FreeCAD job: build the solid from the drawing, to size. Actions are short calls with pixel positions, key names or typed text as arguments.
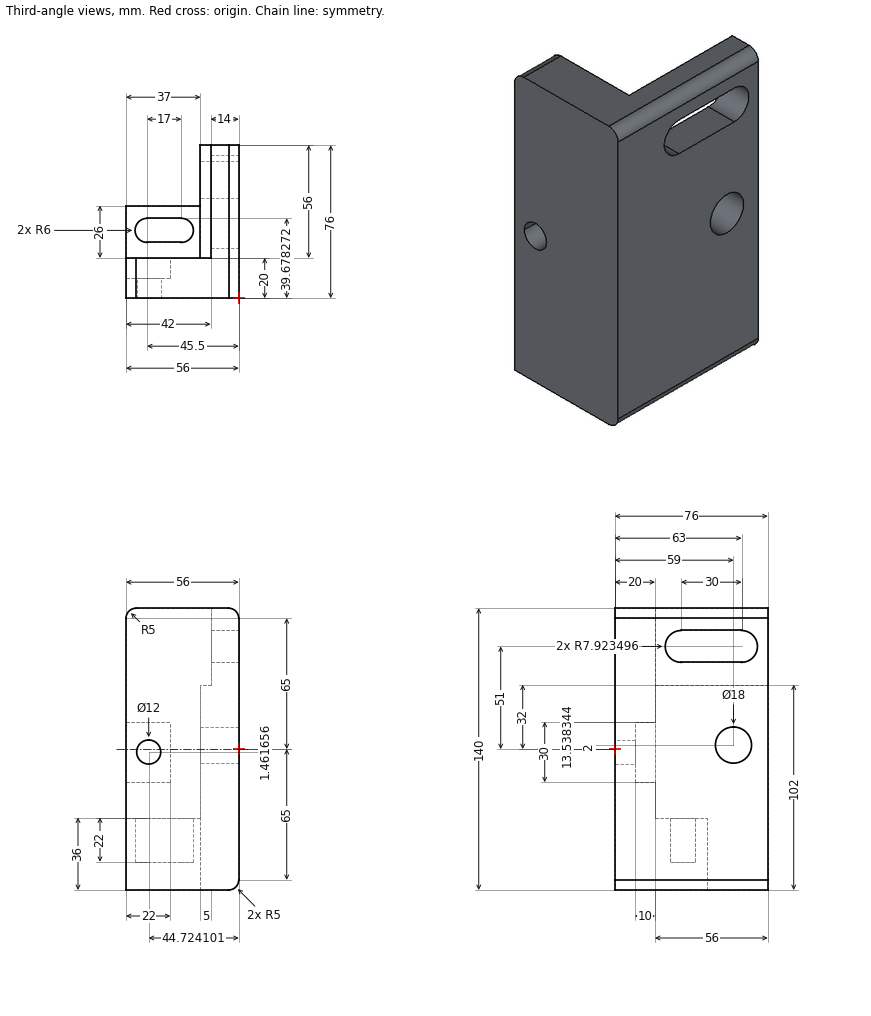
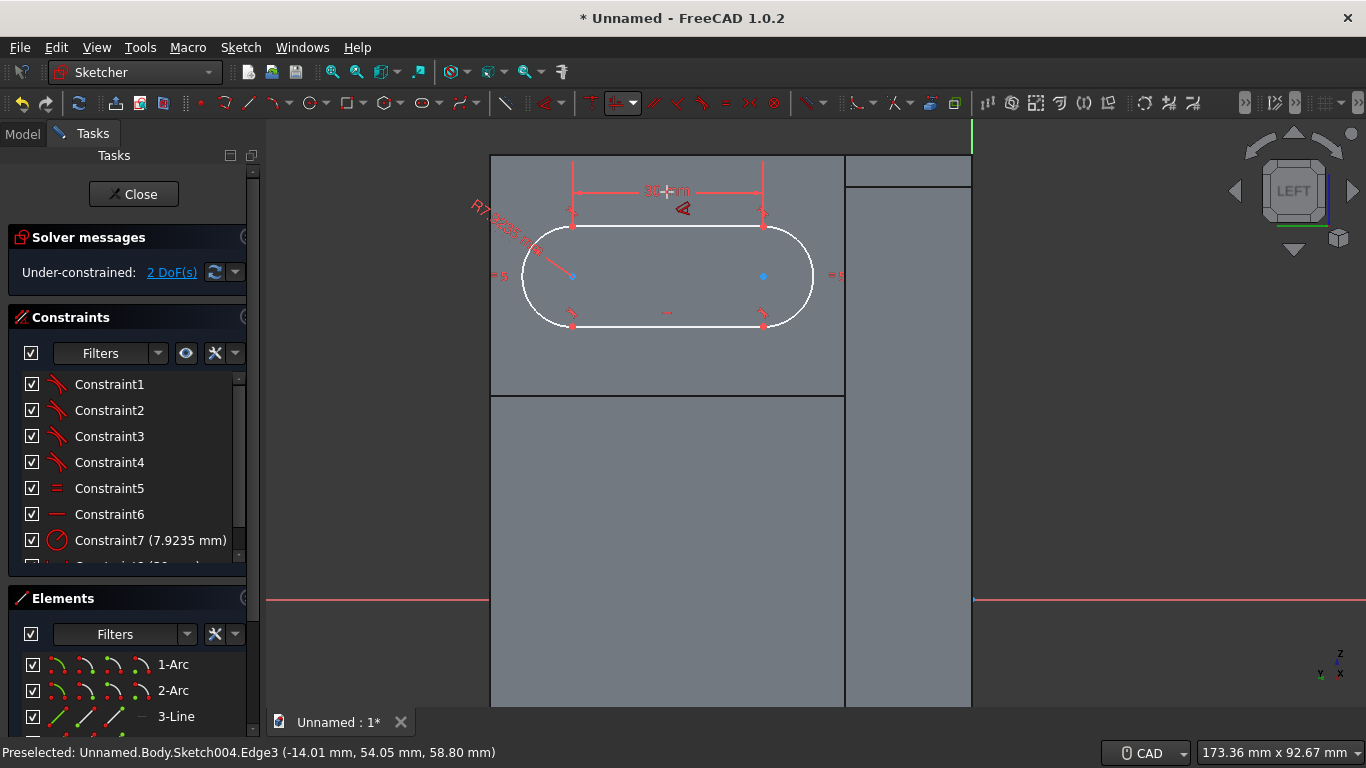
click(573, 226)
click(772, 634)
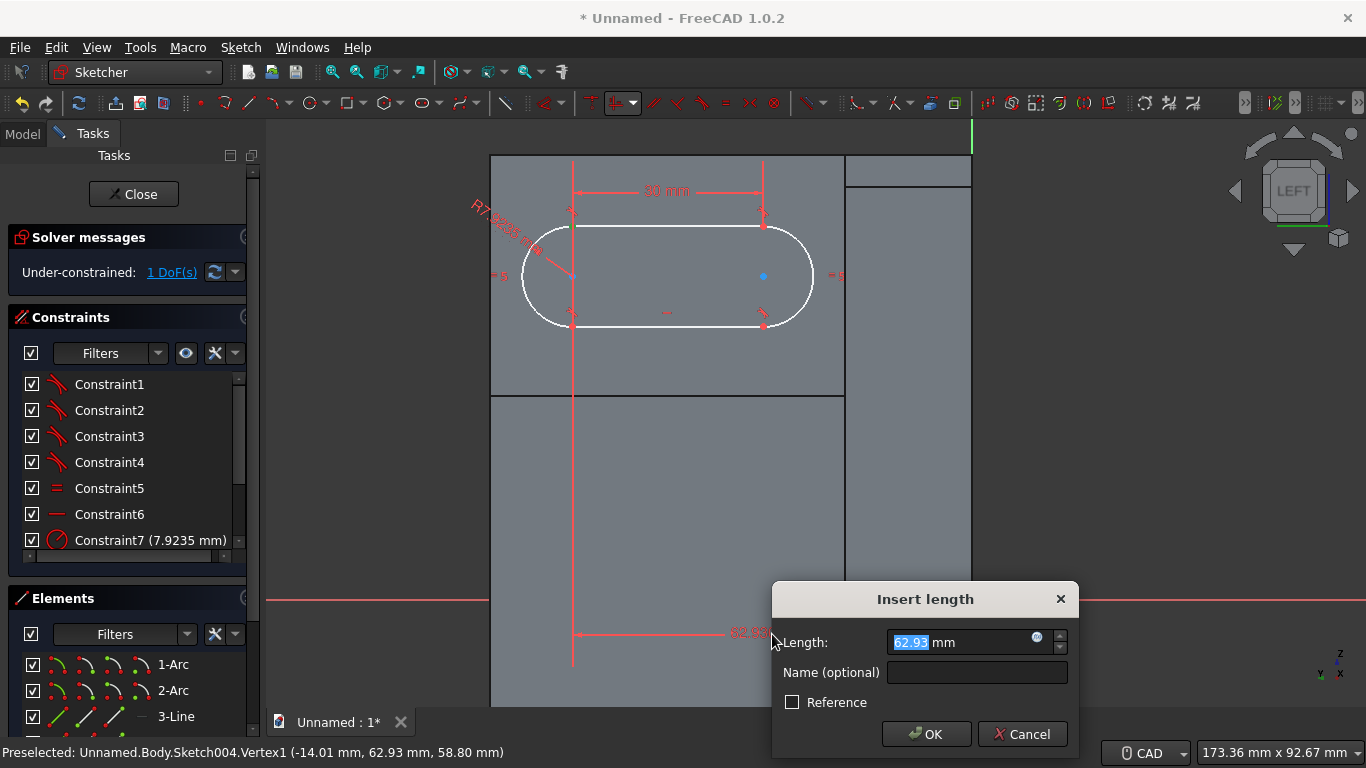
text(63)
key(Return)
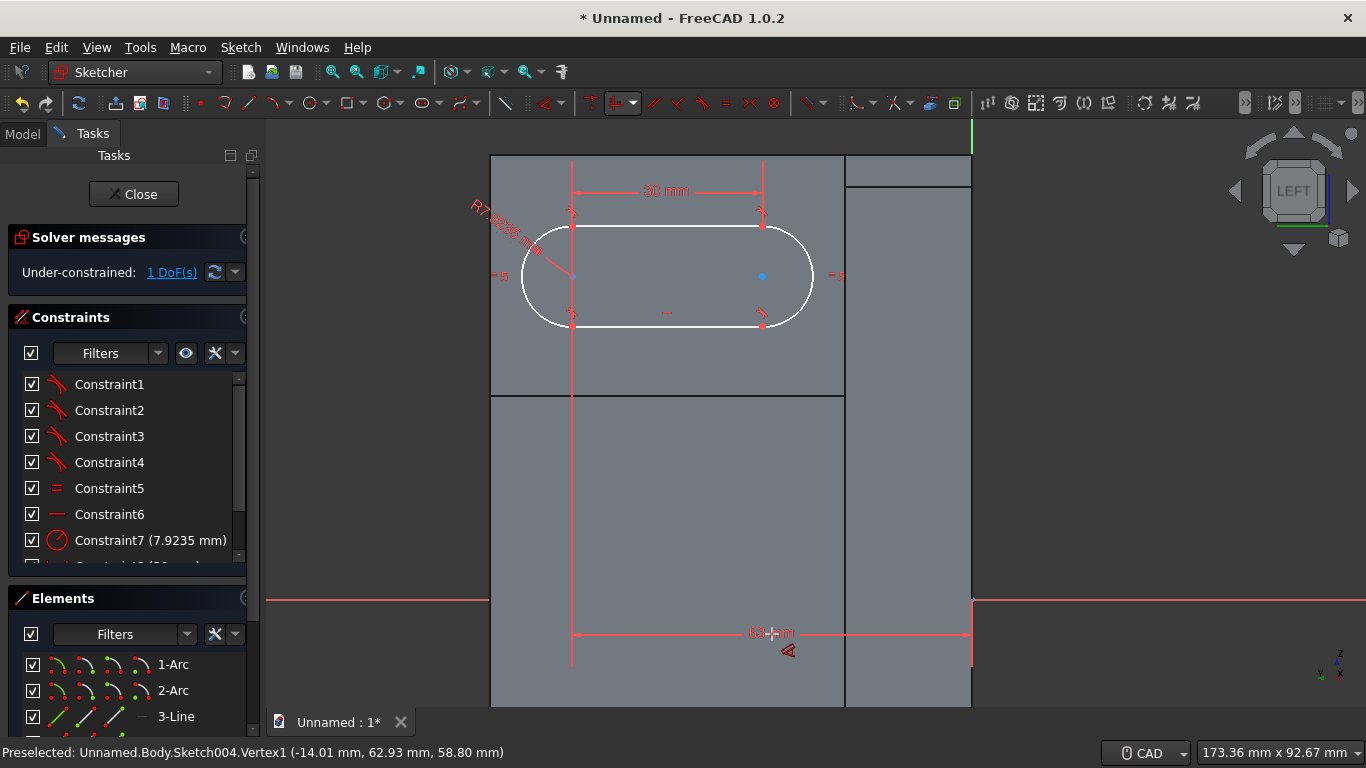
click(572, 277)
click(1006, 438)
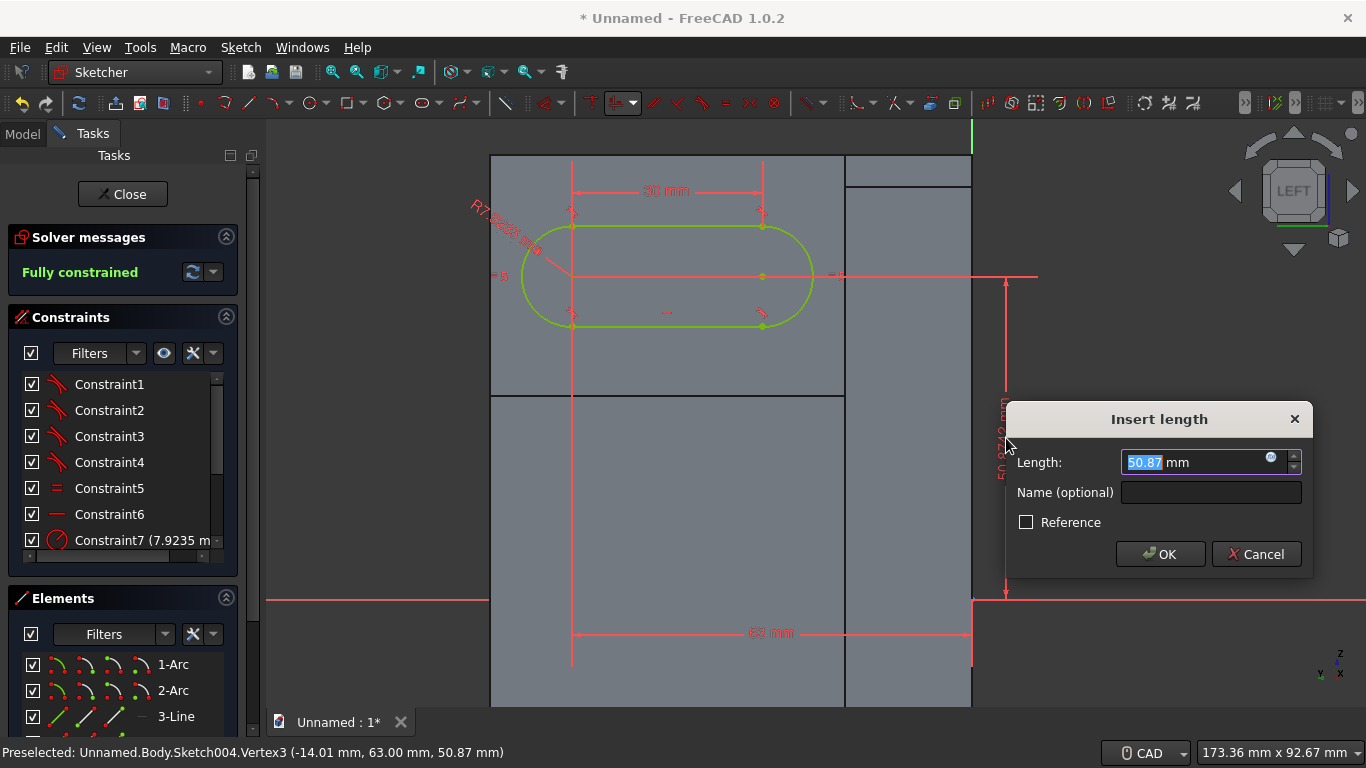
text(51)
key(Return)
key(Escape)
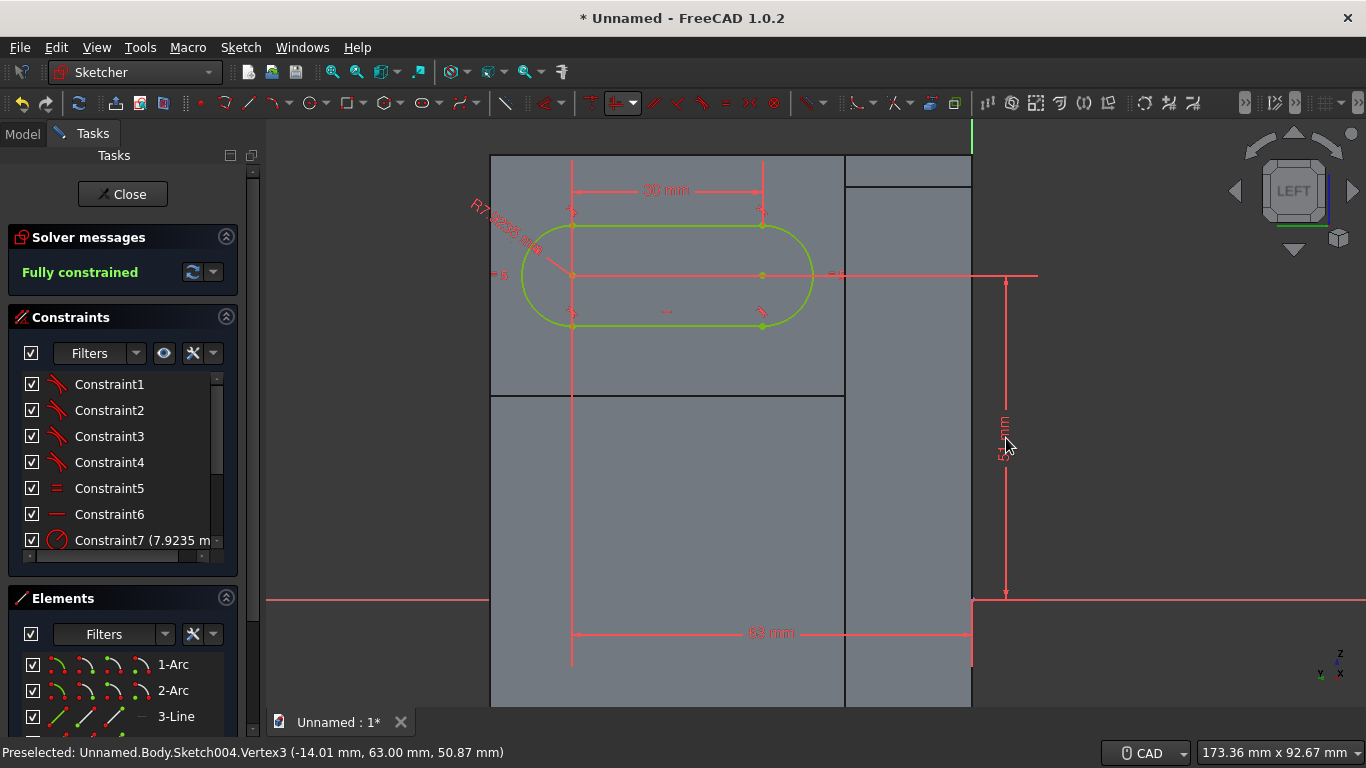
click(123, 194)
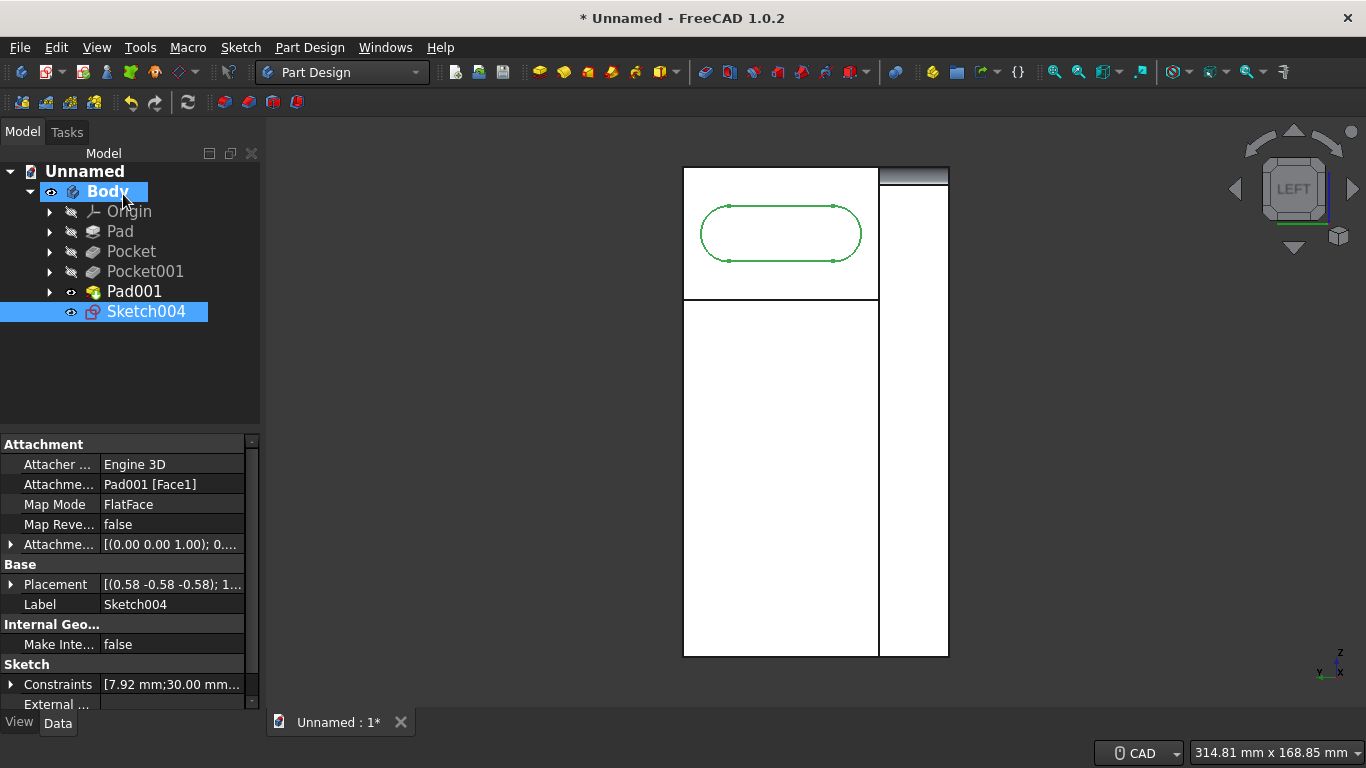
click(706, 72)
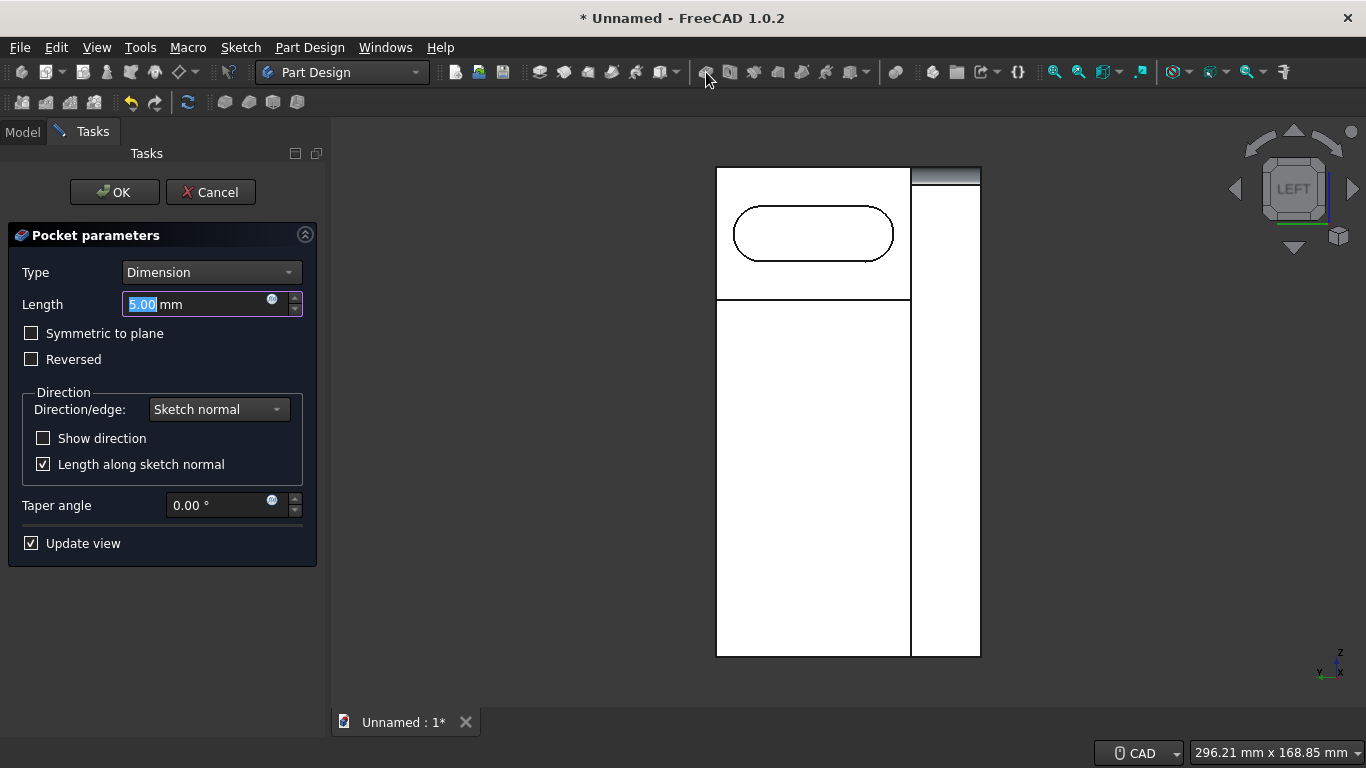
click(212, 272)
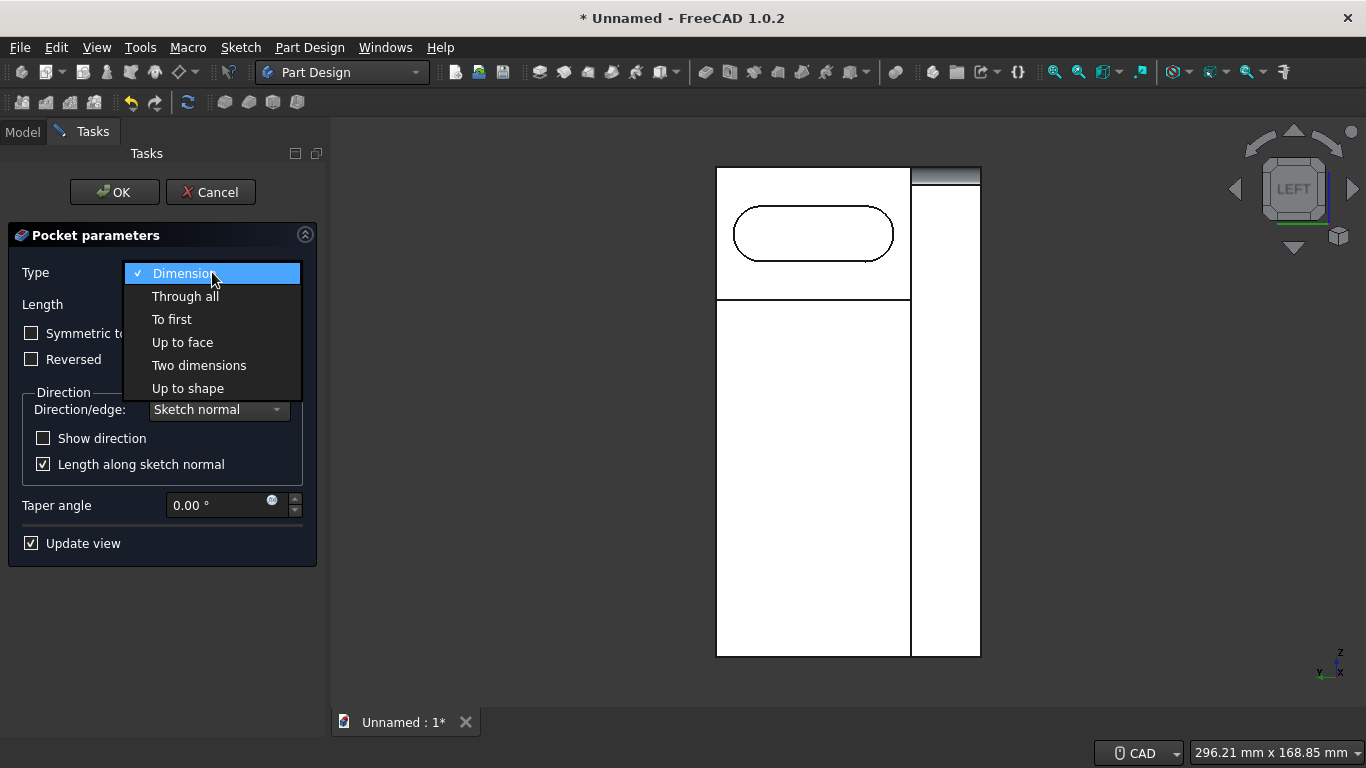
click(212, 296)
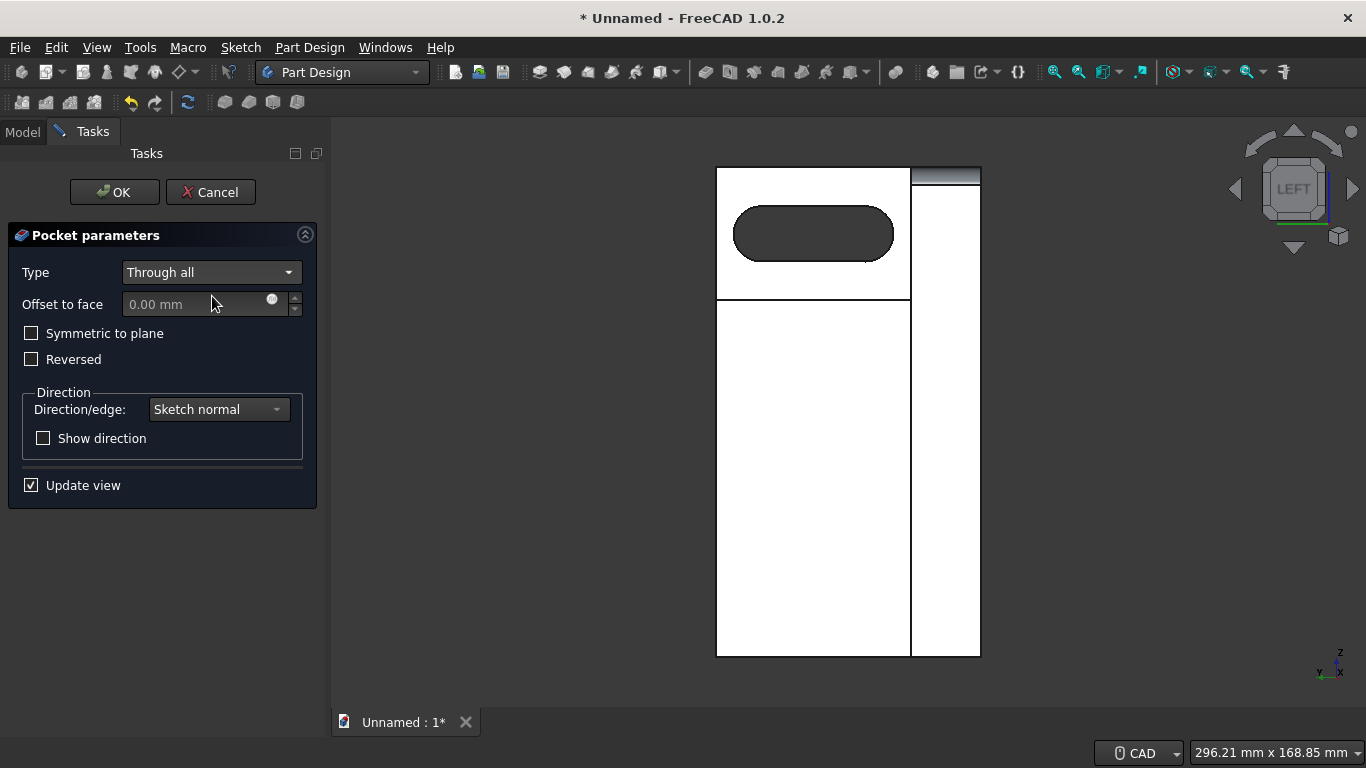
click(115, 192)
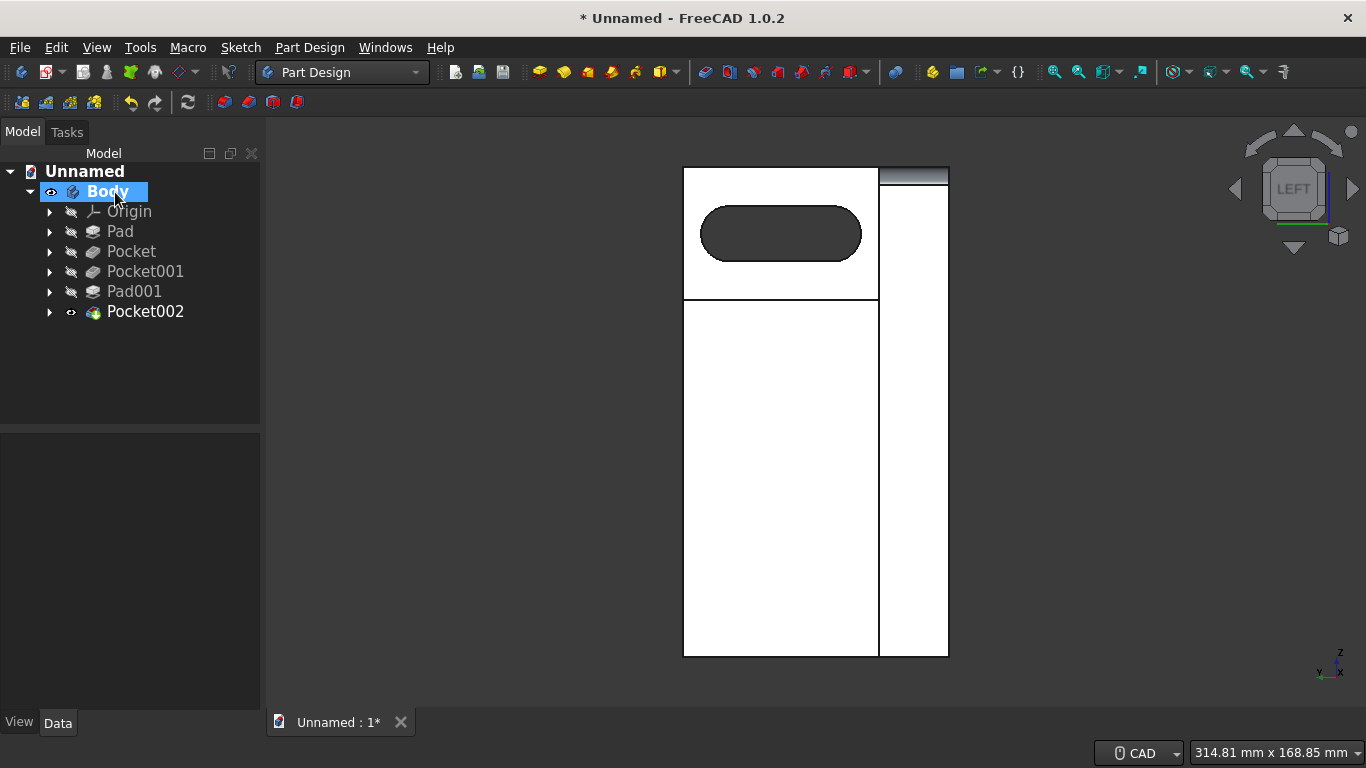
click(781, 426)